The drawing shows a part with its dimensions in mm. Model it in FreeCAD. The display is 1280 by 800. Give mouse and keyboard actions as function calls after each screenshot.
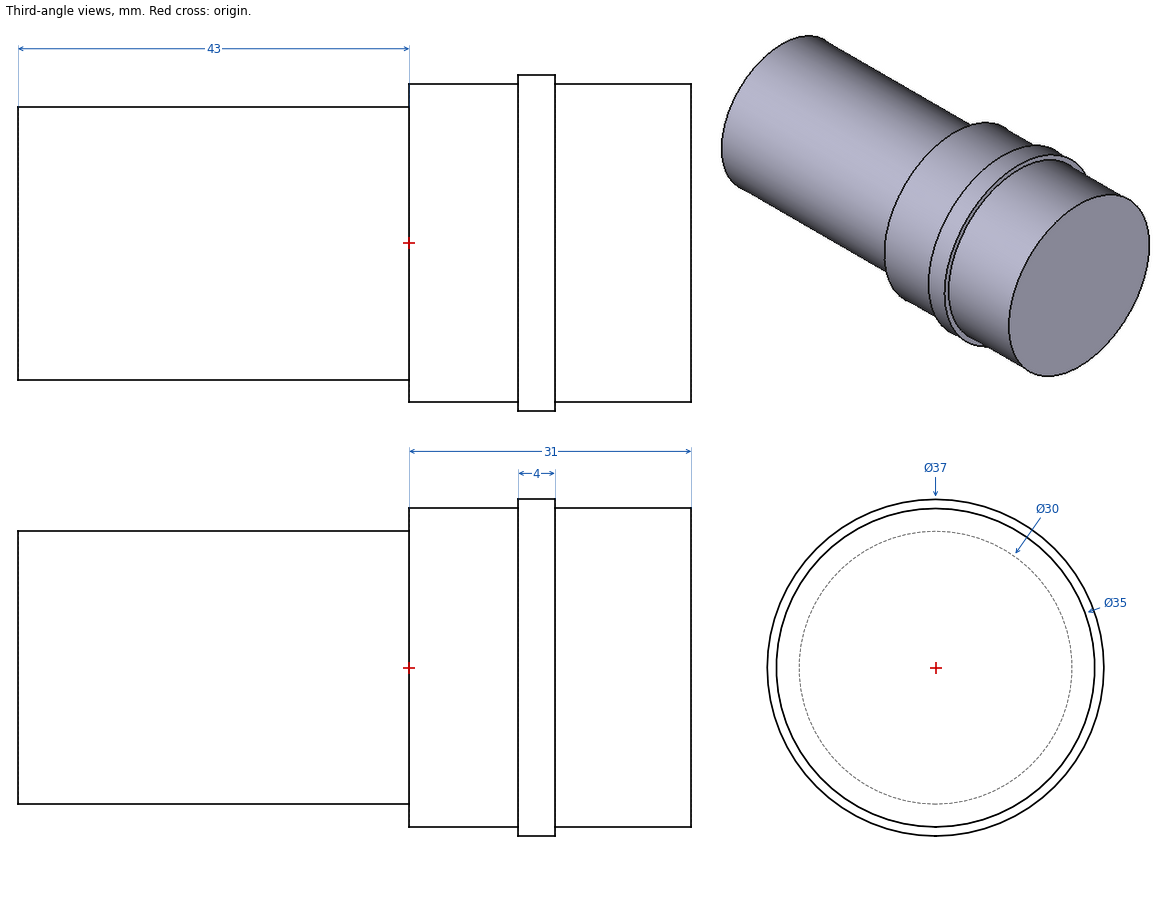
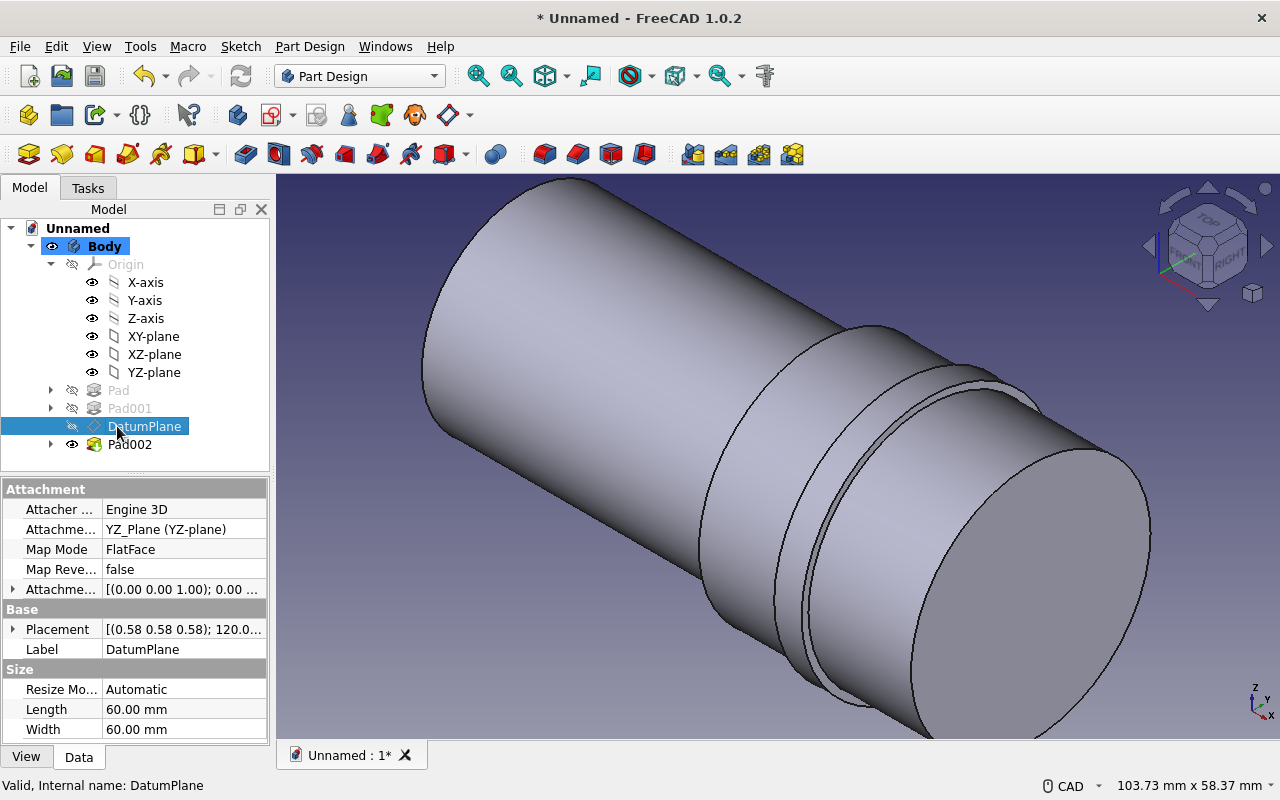
click(479, 76)